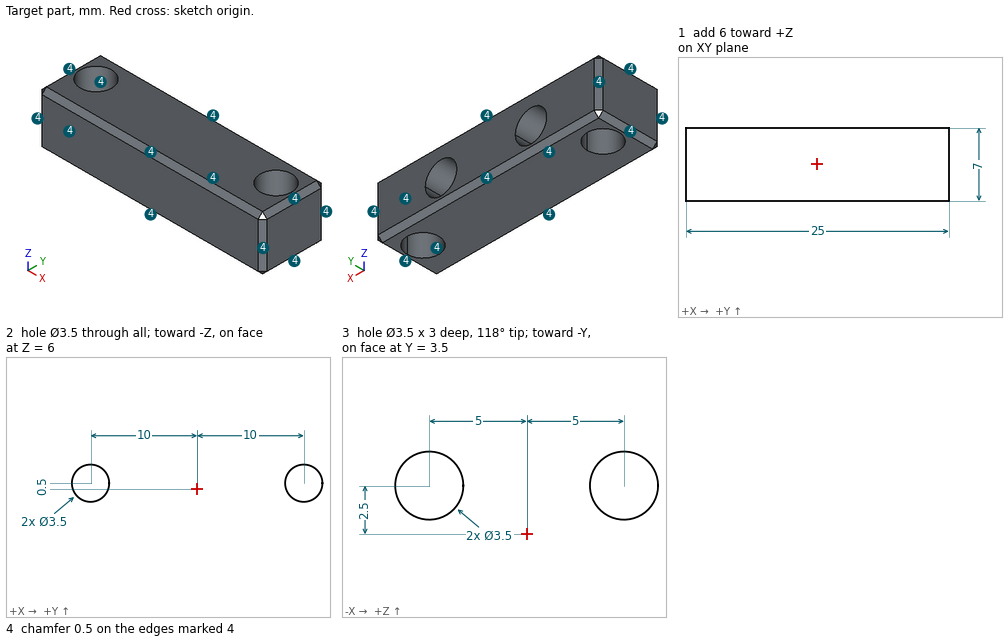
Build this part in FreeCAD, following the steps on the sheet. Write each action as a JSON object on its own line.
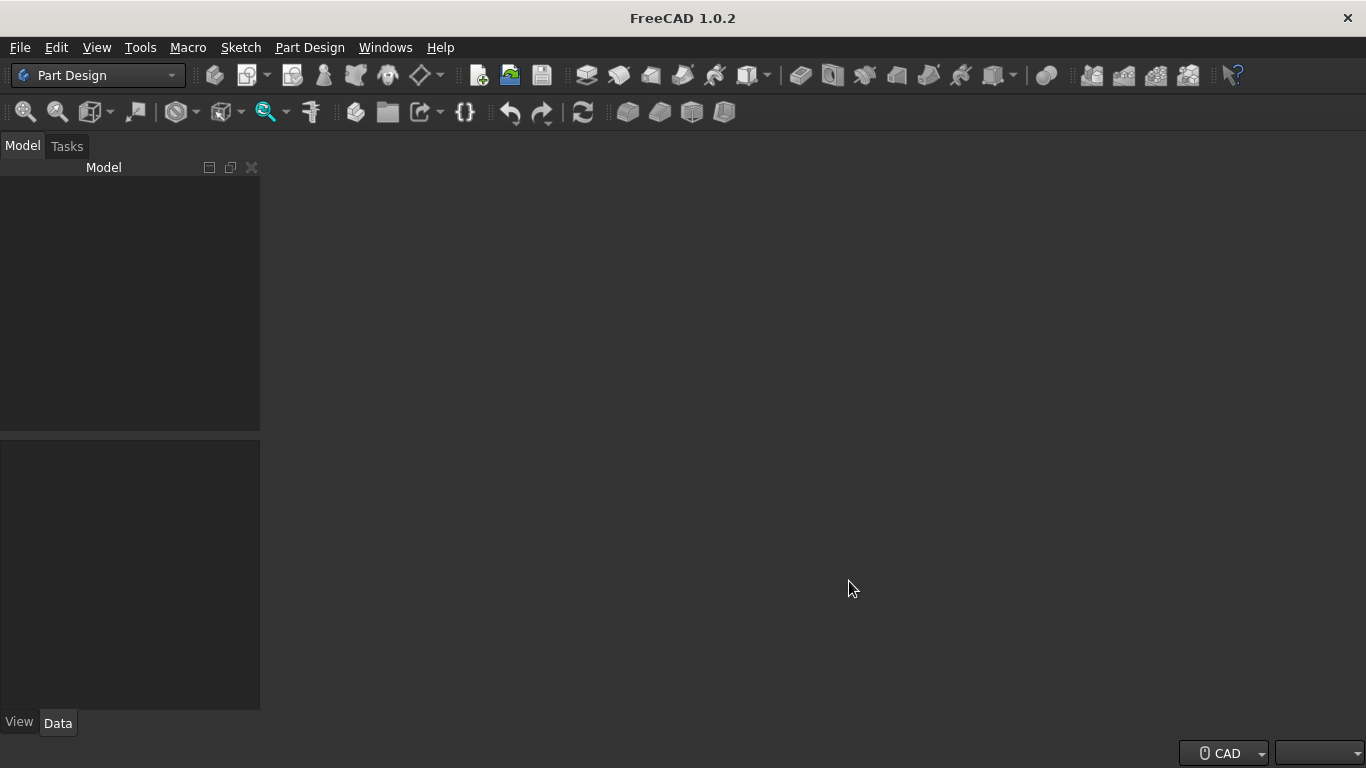
{"action": "left_click", "coordinate": [478, 76]}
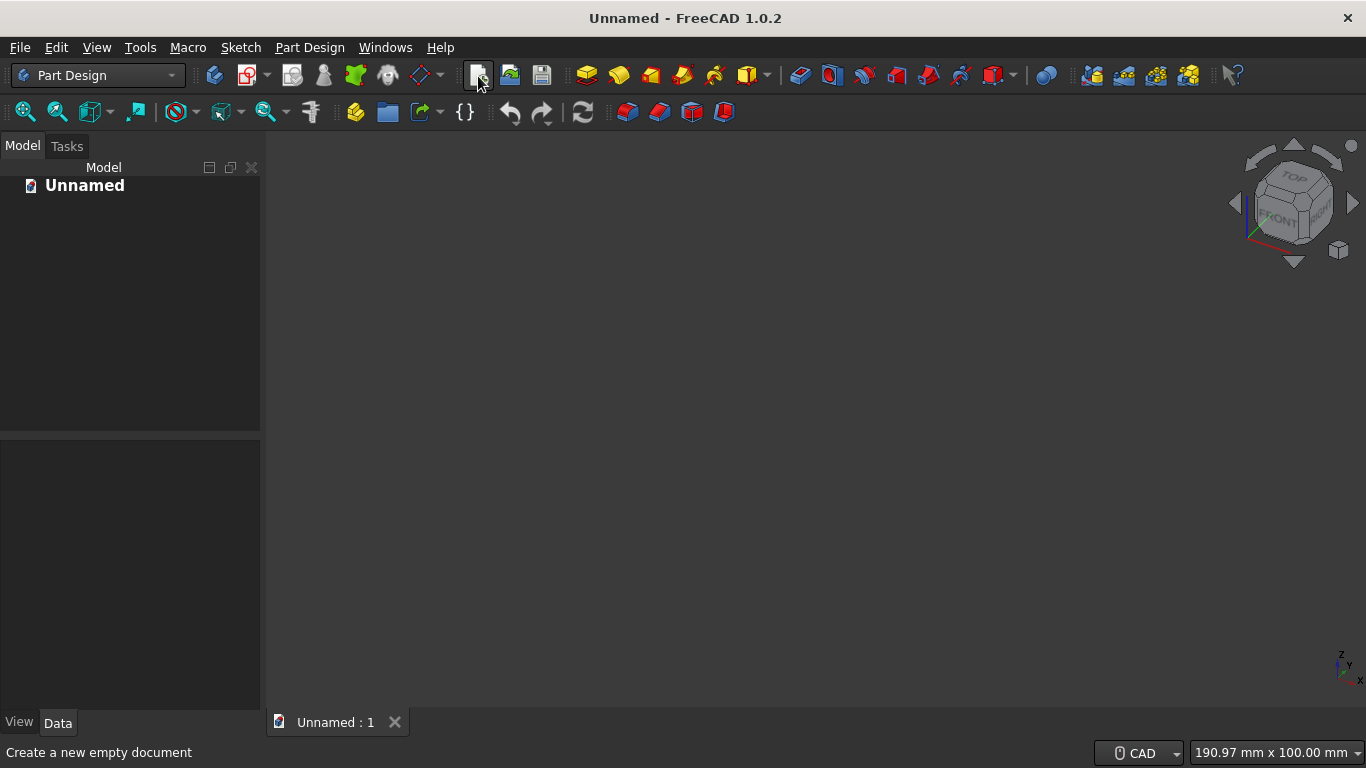
{"action": "left_click", "coordinate": [248, 76]}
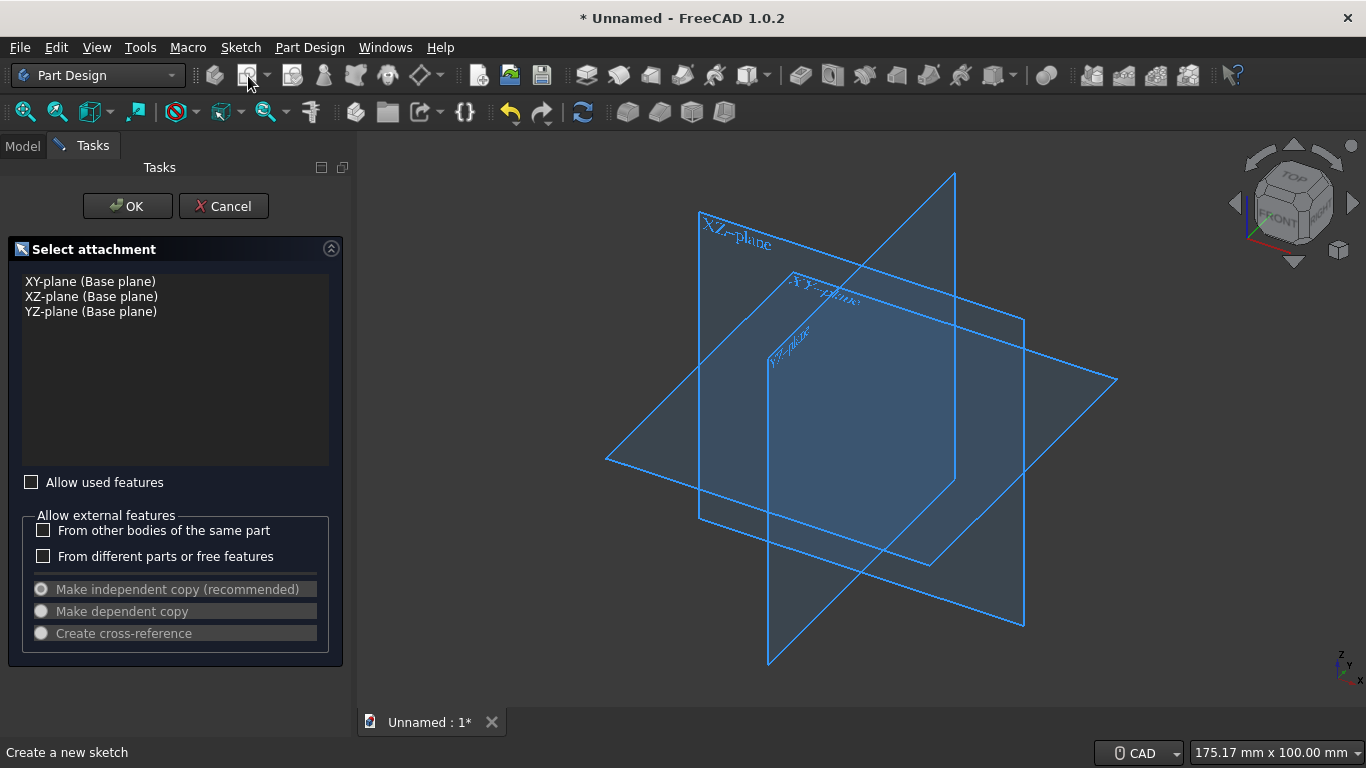
{"action": "left_click", "coordinate": [82, 282]}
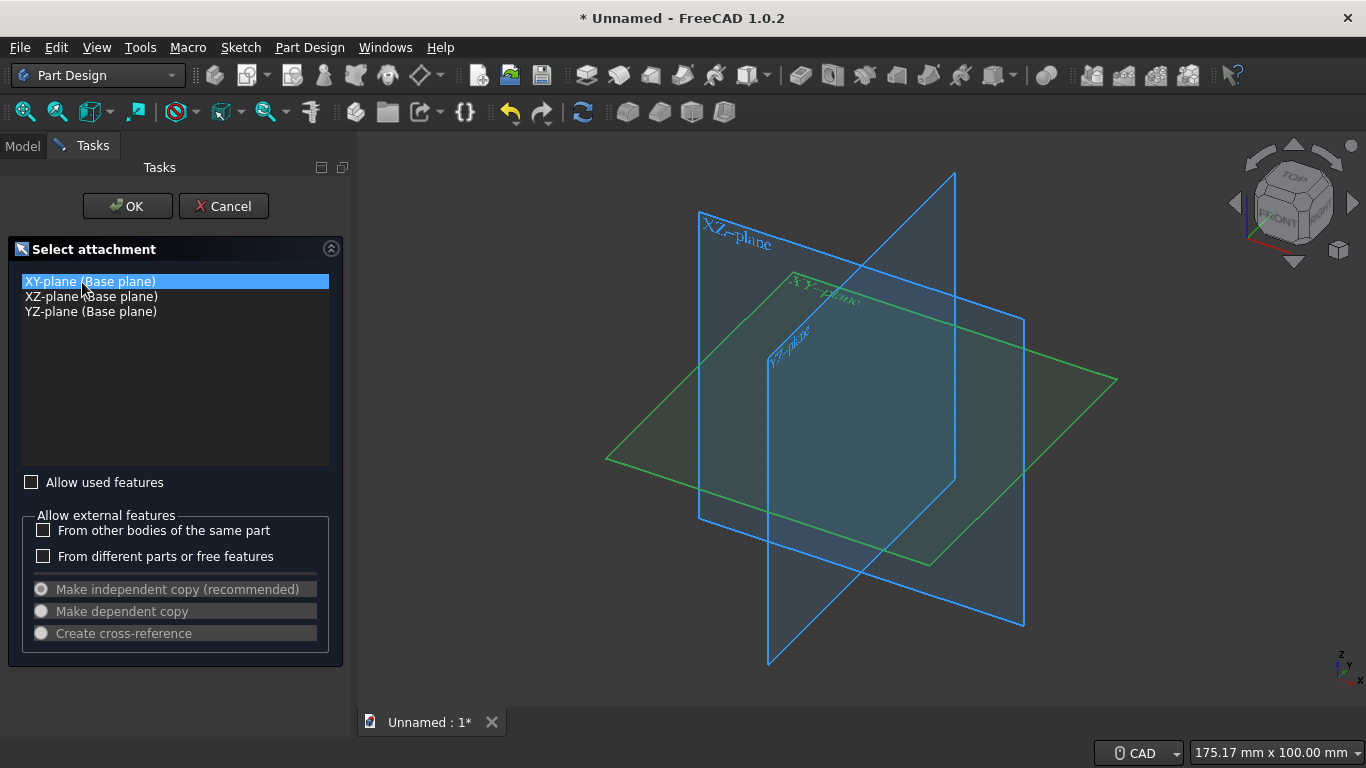
{"action": "left_click", "coordinate": [128, 206]}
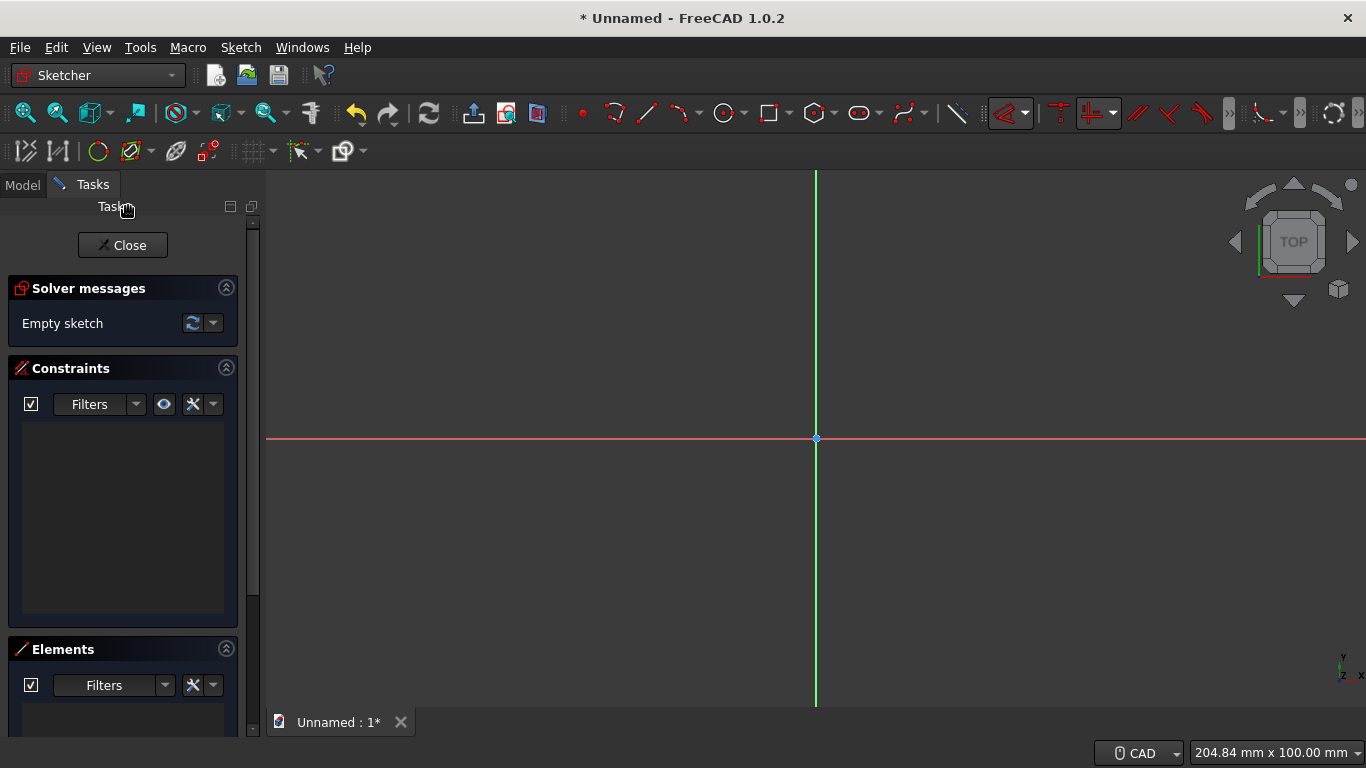
{"action": "scroll", "coordinate": [833, 438], "scroll_direction": "up", "scroll_amount": 8}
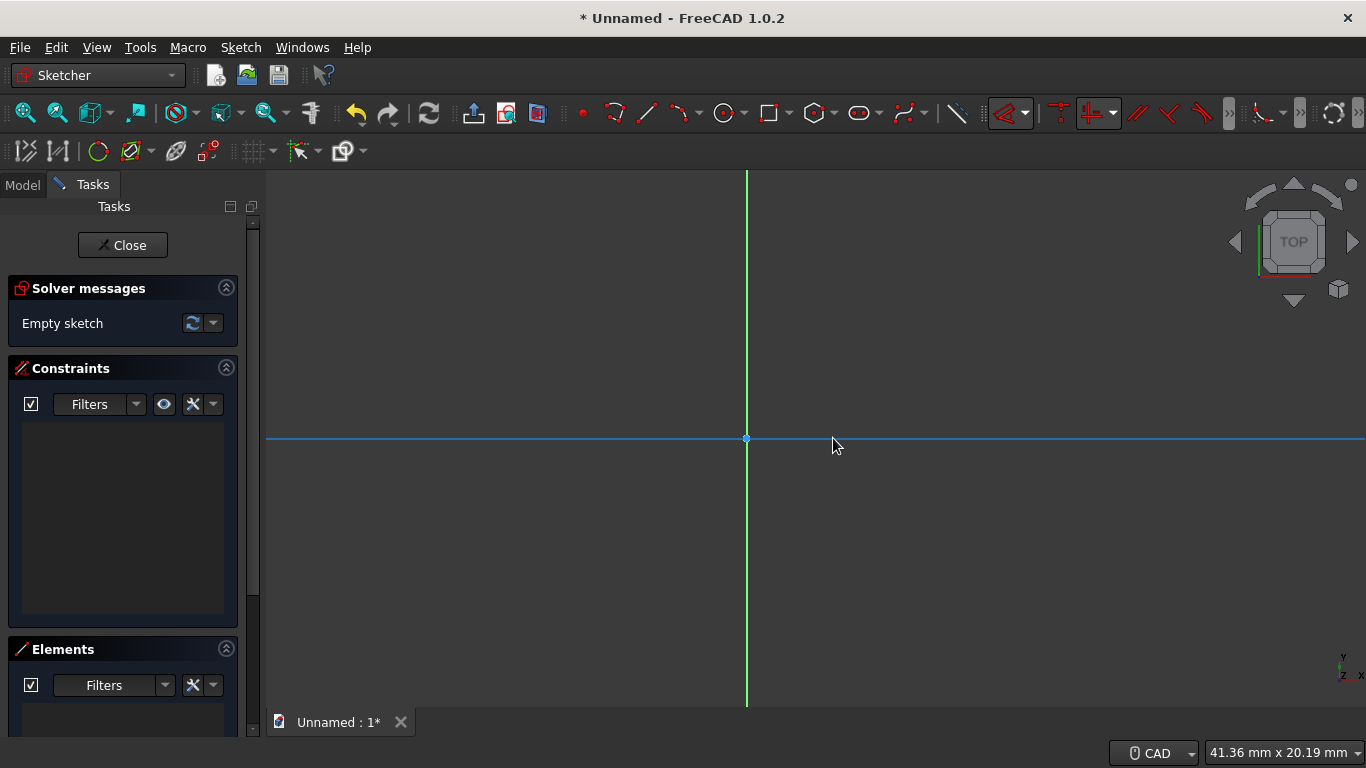
{"action": "key", "text": "g v"}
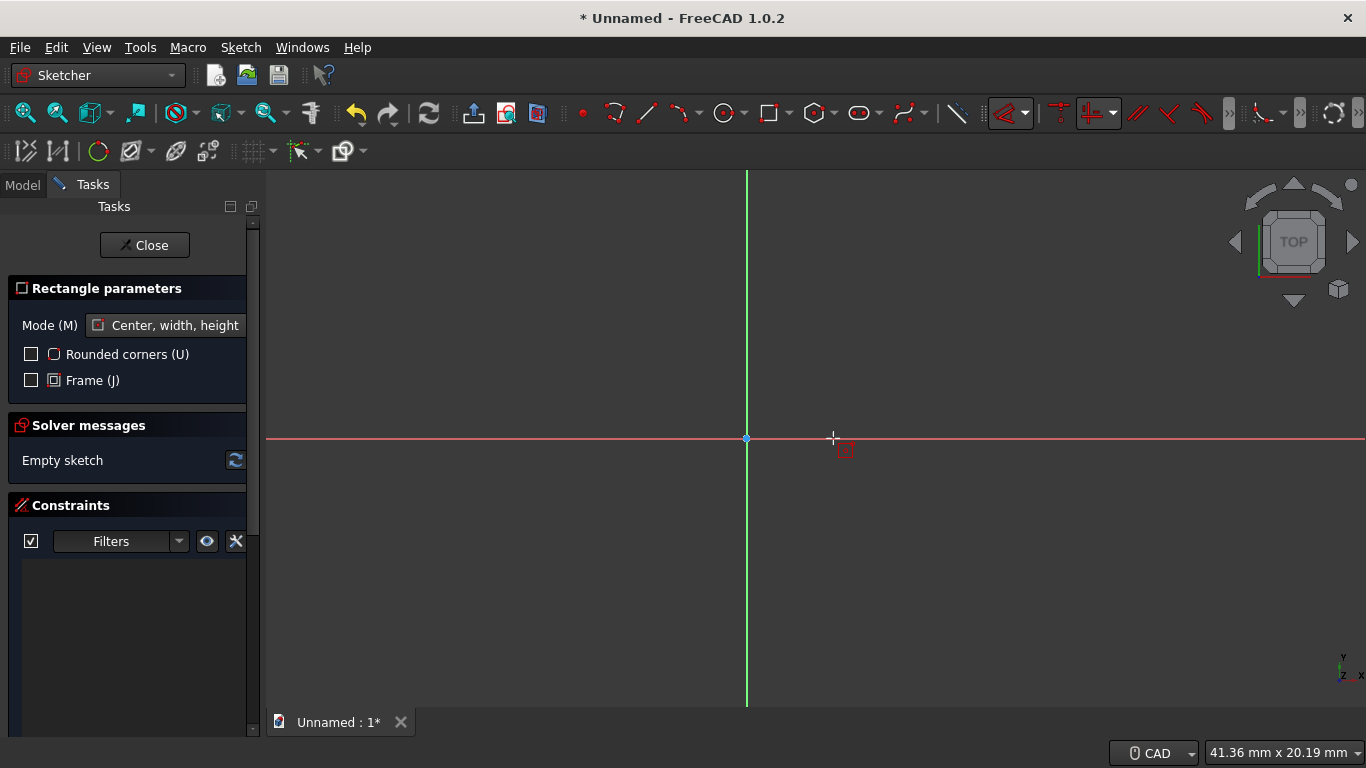
{"action": "left_click", "coordinate": [747, 438]}
{"action": "mouse_move", "coordinate": [1079, 345]}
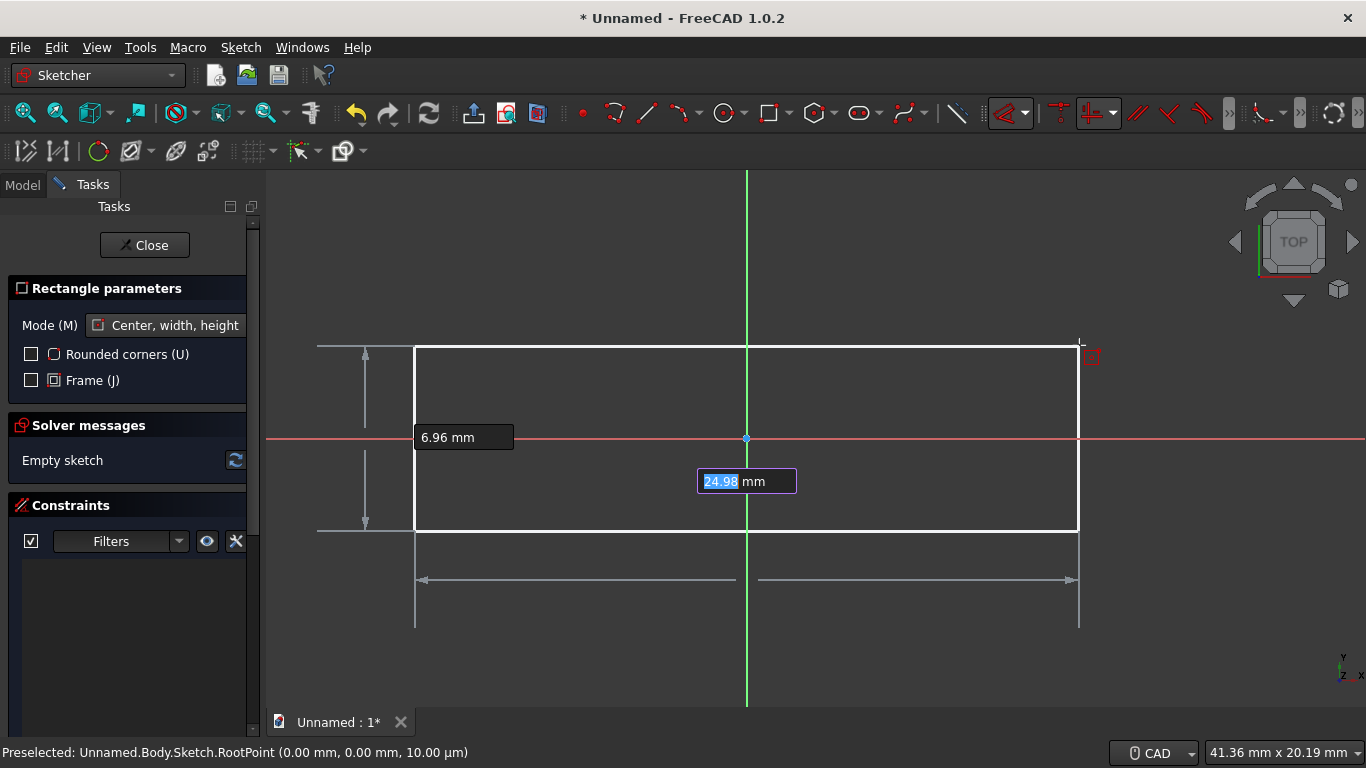
{"action": "type", "text": "25"}
{"action": "key", "text": "Tab"}
{"action": "type", "text": "7"}
{"action": "key", "text": "Return"}
{"action": "key", "text": "Escape"}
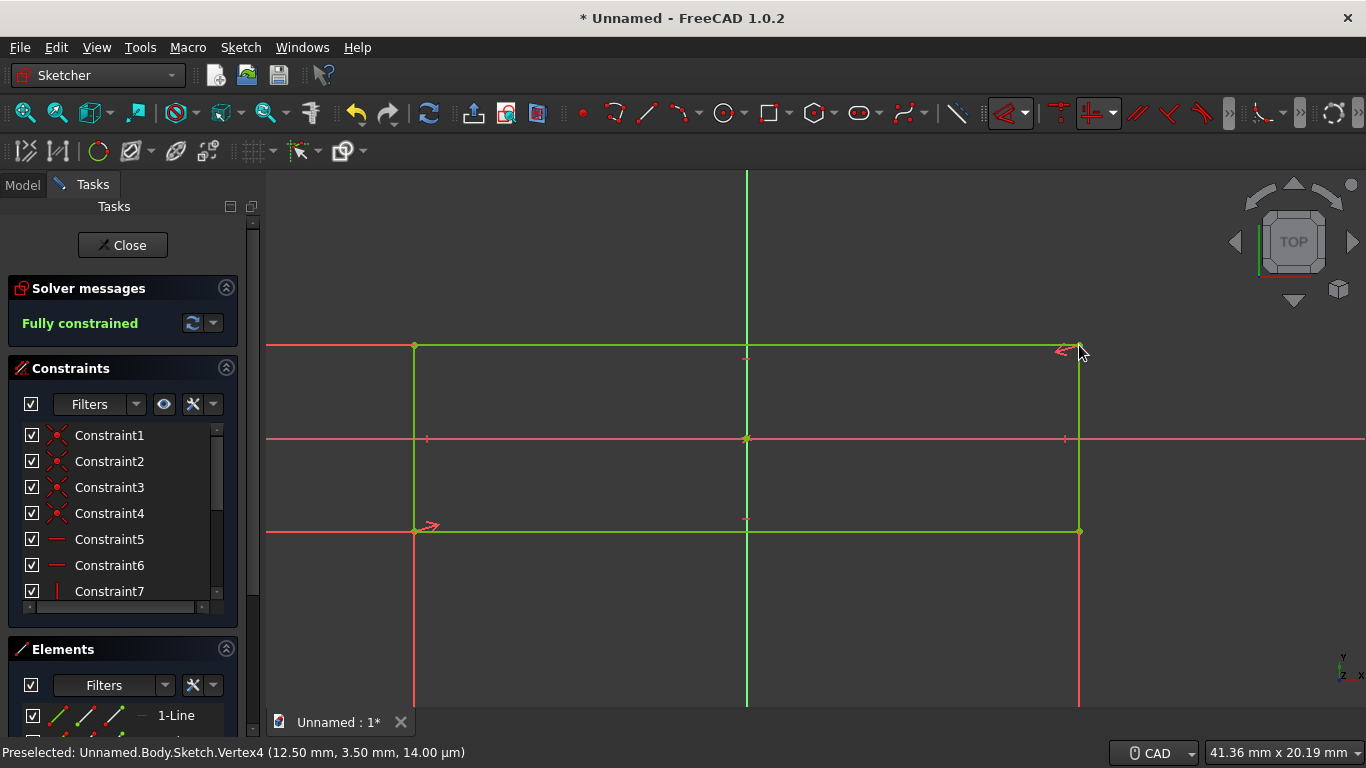
{"action": "left_click", "coordinate": [123, 245]}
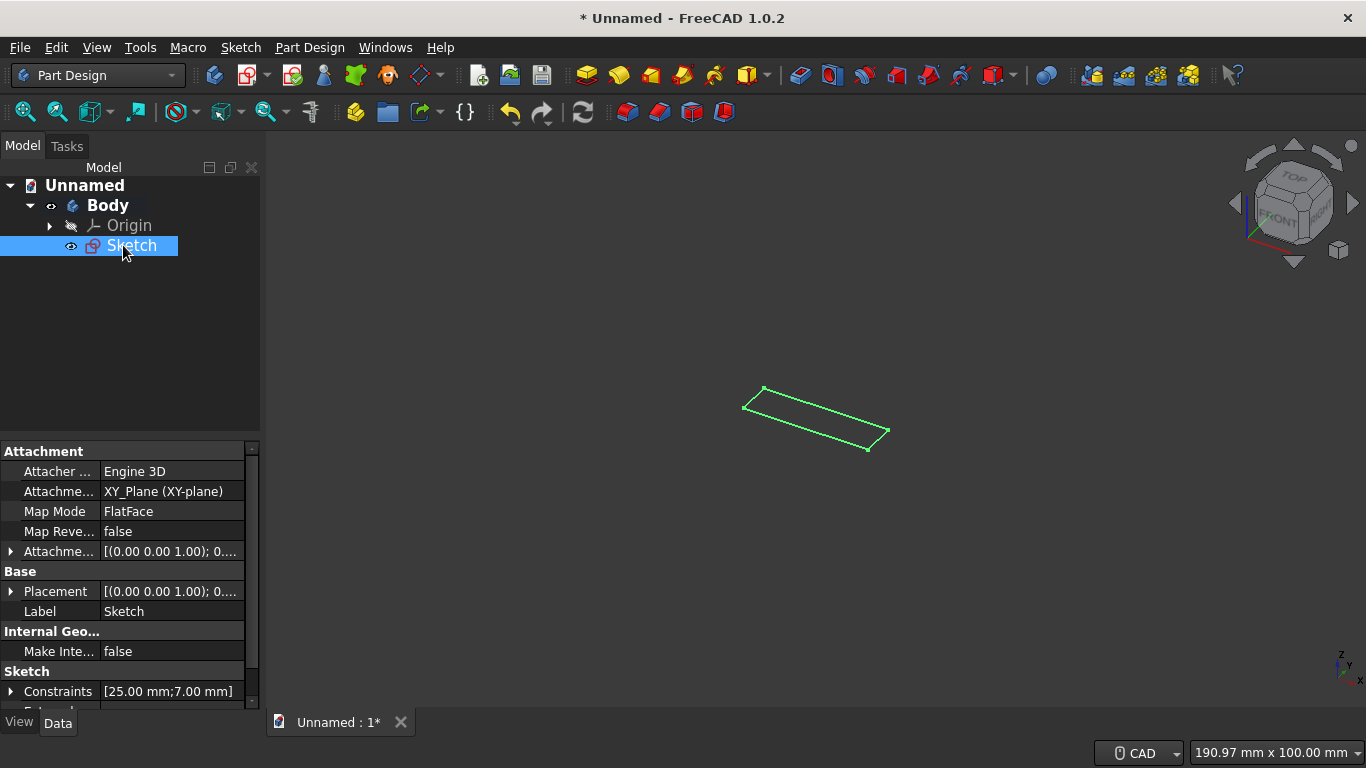
{"action": "left_click", "coordinate": [588, 76]}